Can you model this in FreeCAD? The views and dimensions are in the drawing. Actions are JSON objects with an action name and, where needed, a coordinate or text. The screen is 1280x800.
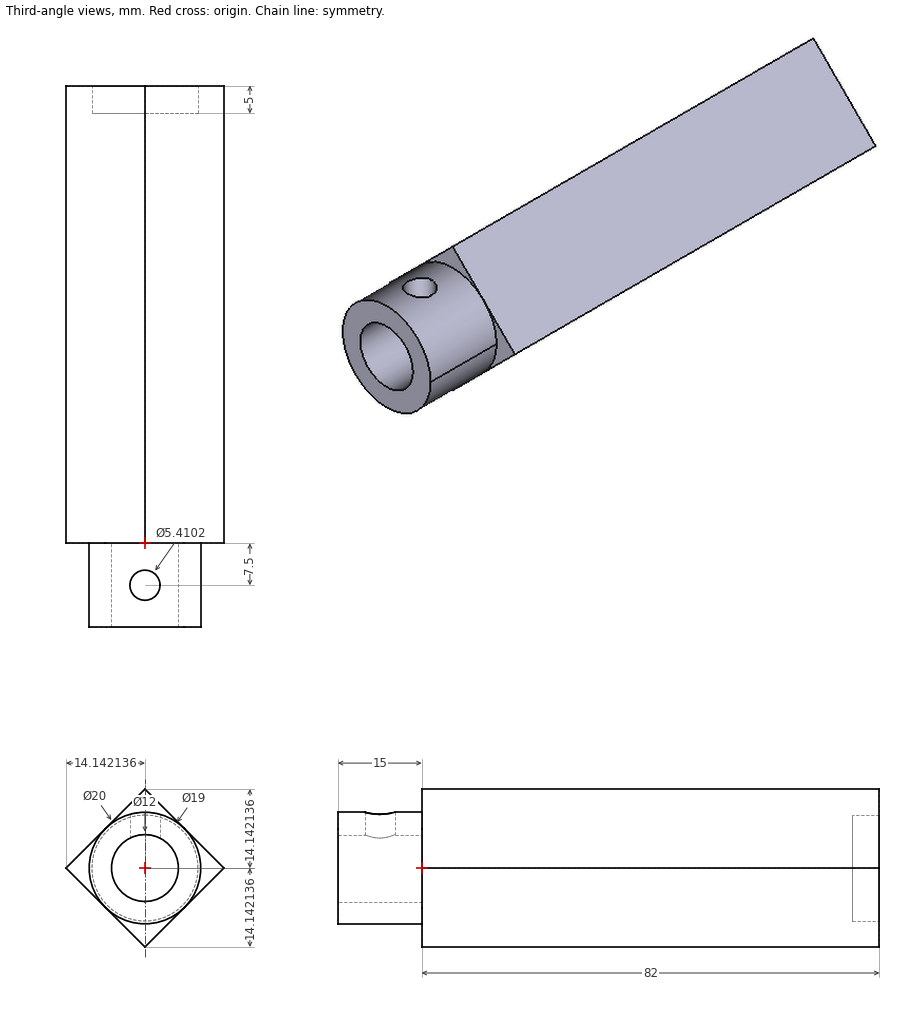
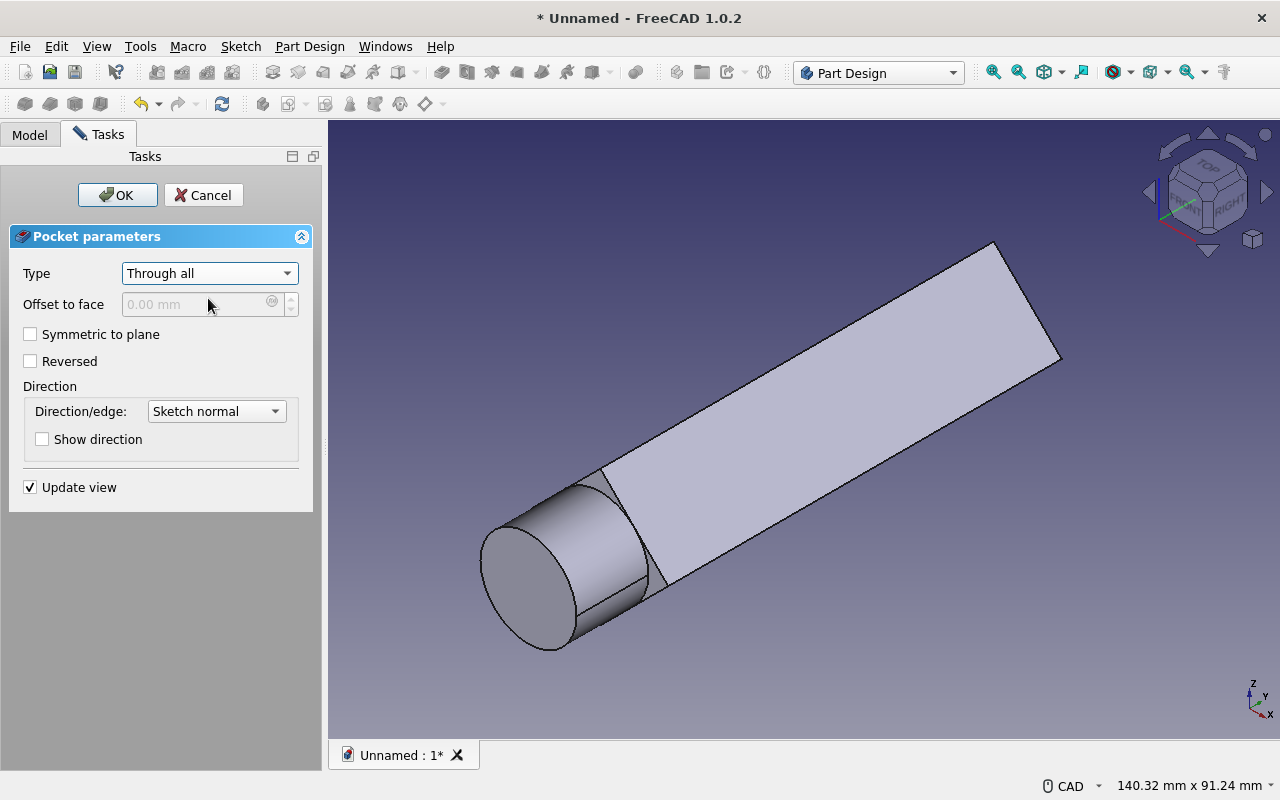
{"action": "left_click", "coordinate": [31, 361]}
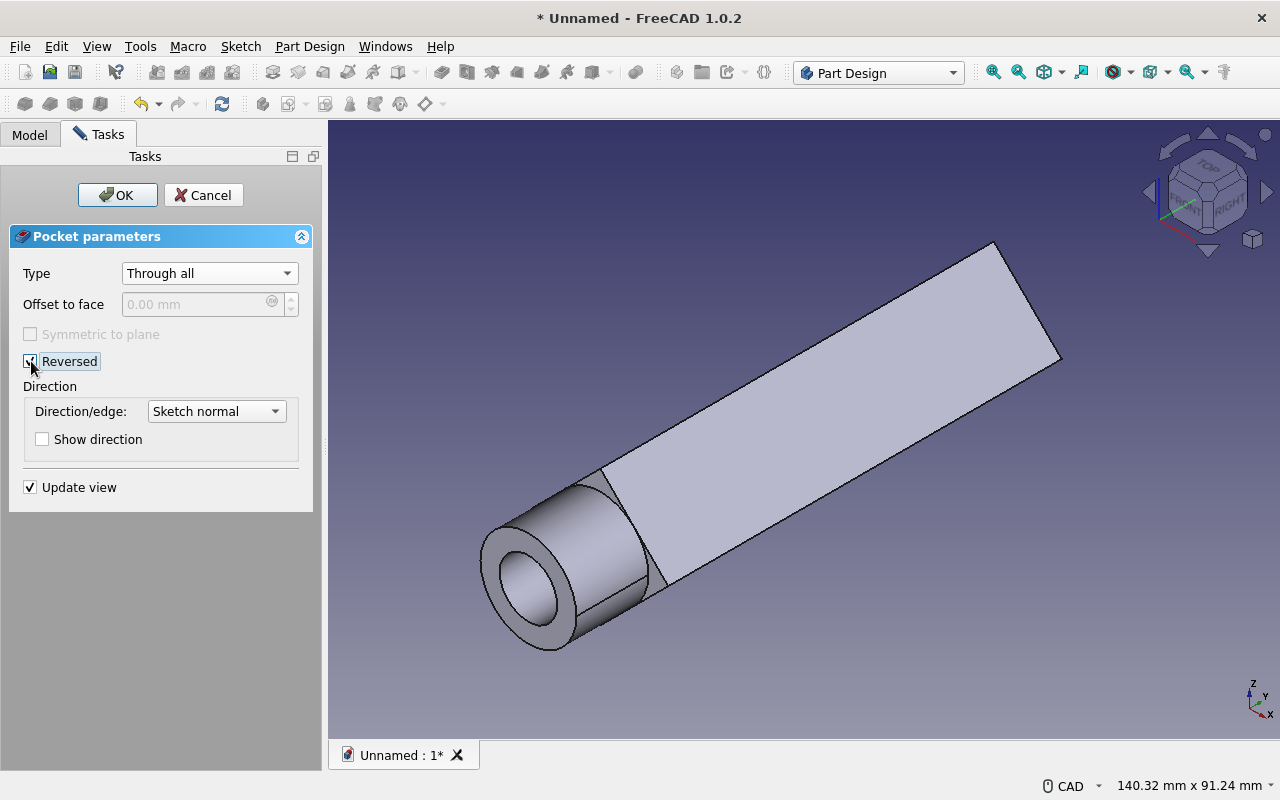
{"action": "left_click", "coordinate": [118, 195]}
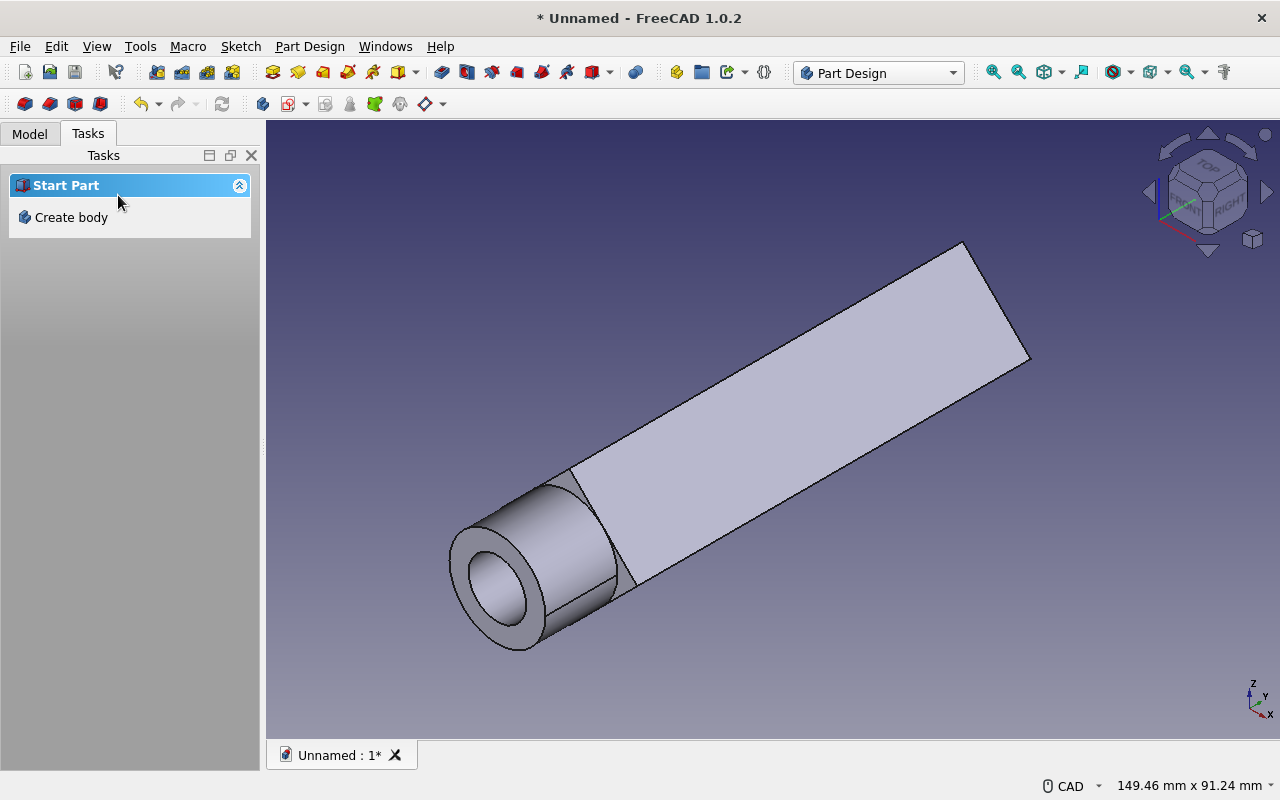
{"action": "left_click", "coordinate": [30, 134]}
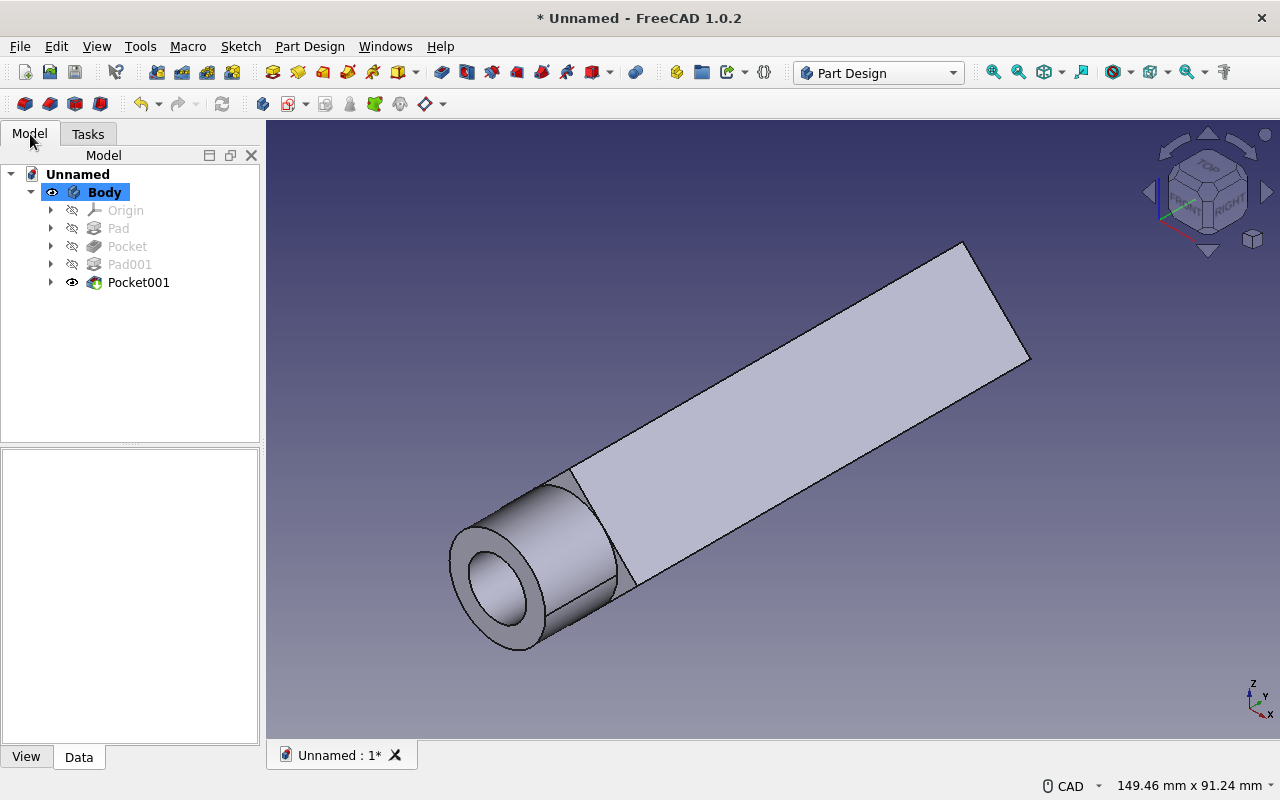
{"action": "left_click", "coordinate": [51, 210]}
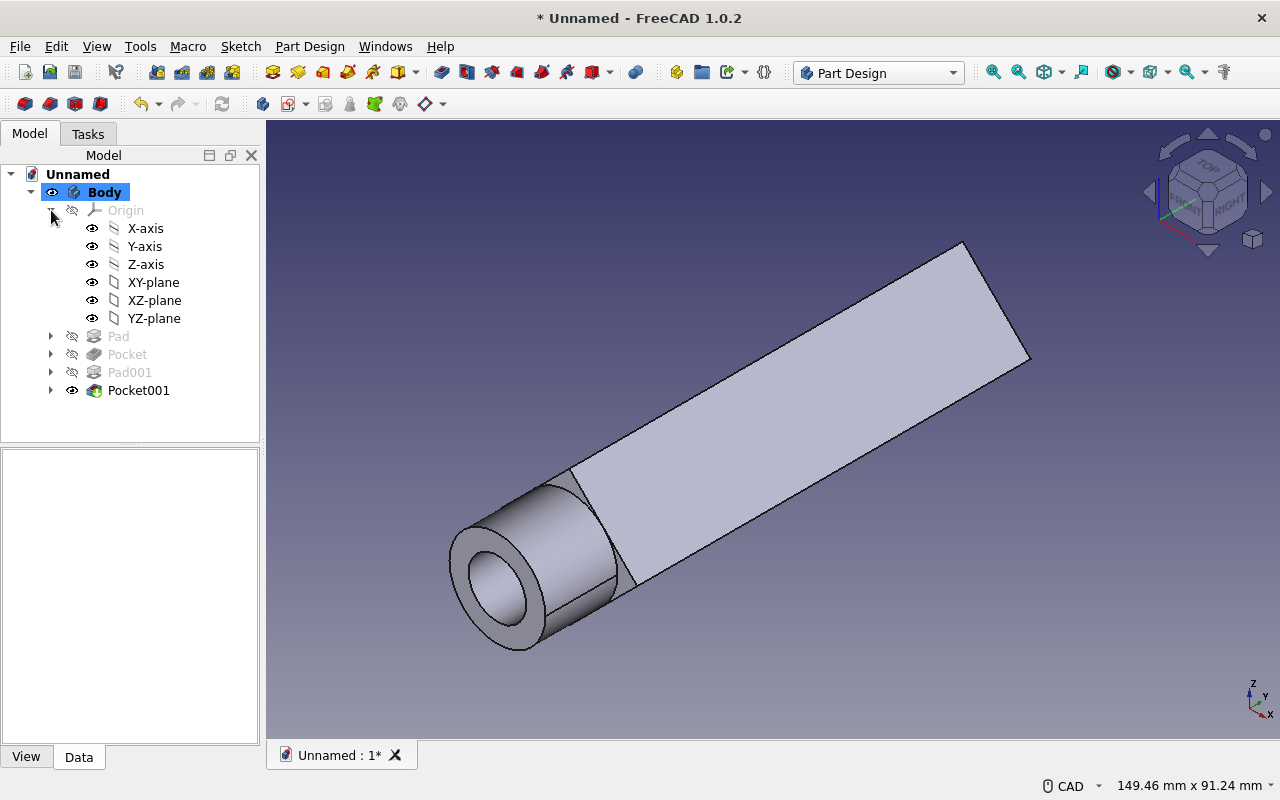
{"action": "left_click", "coordinate": [137, 282]}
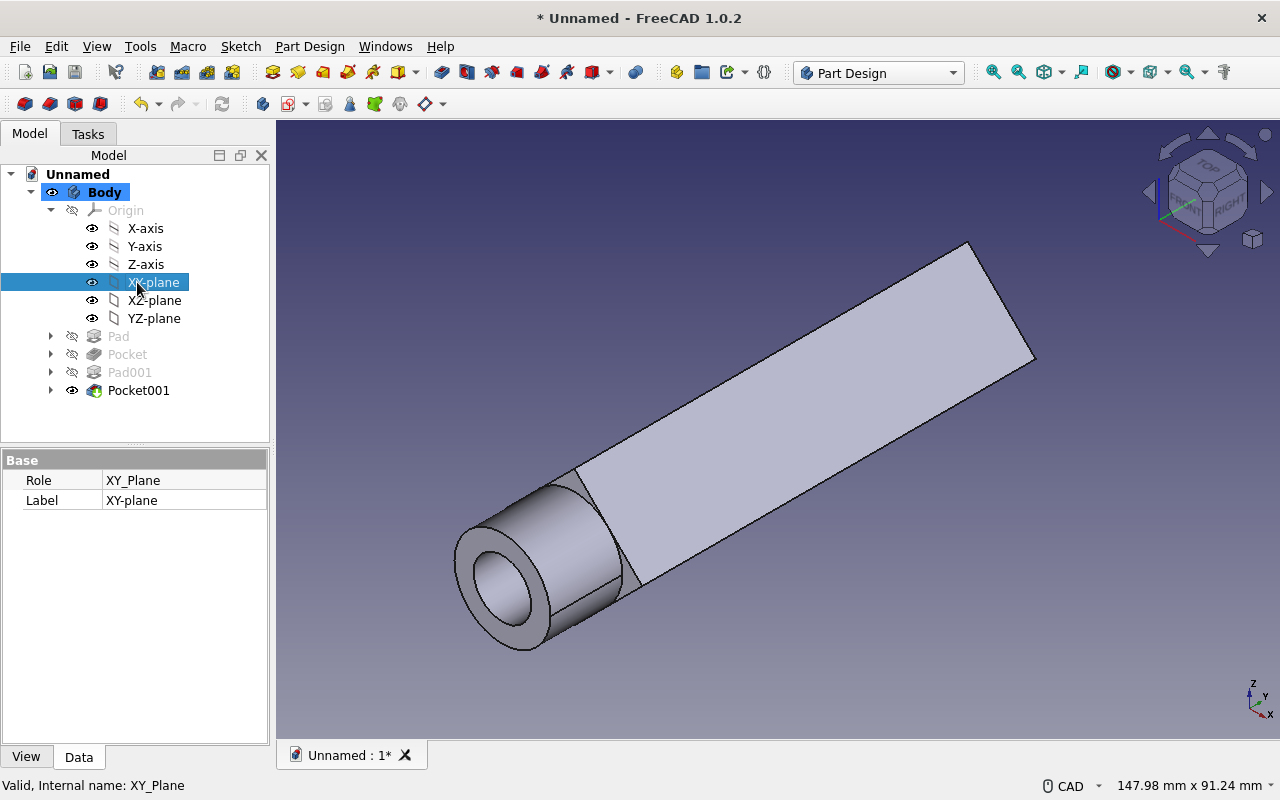
{"action": "left_click", "coordinate": [424, 104]}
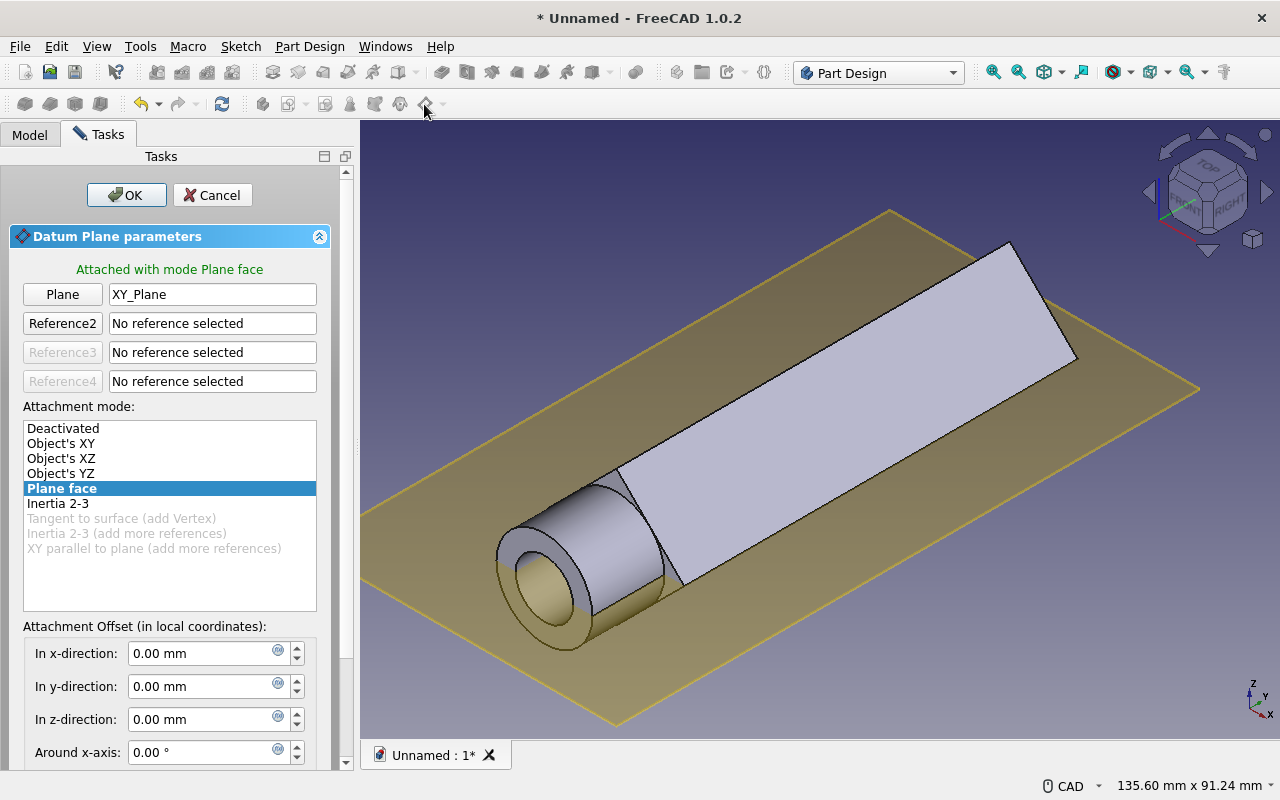
{"action": "triple_click", "coordinate": [210, 720]}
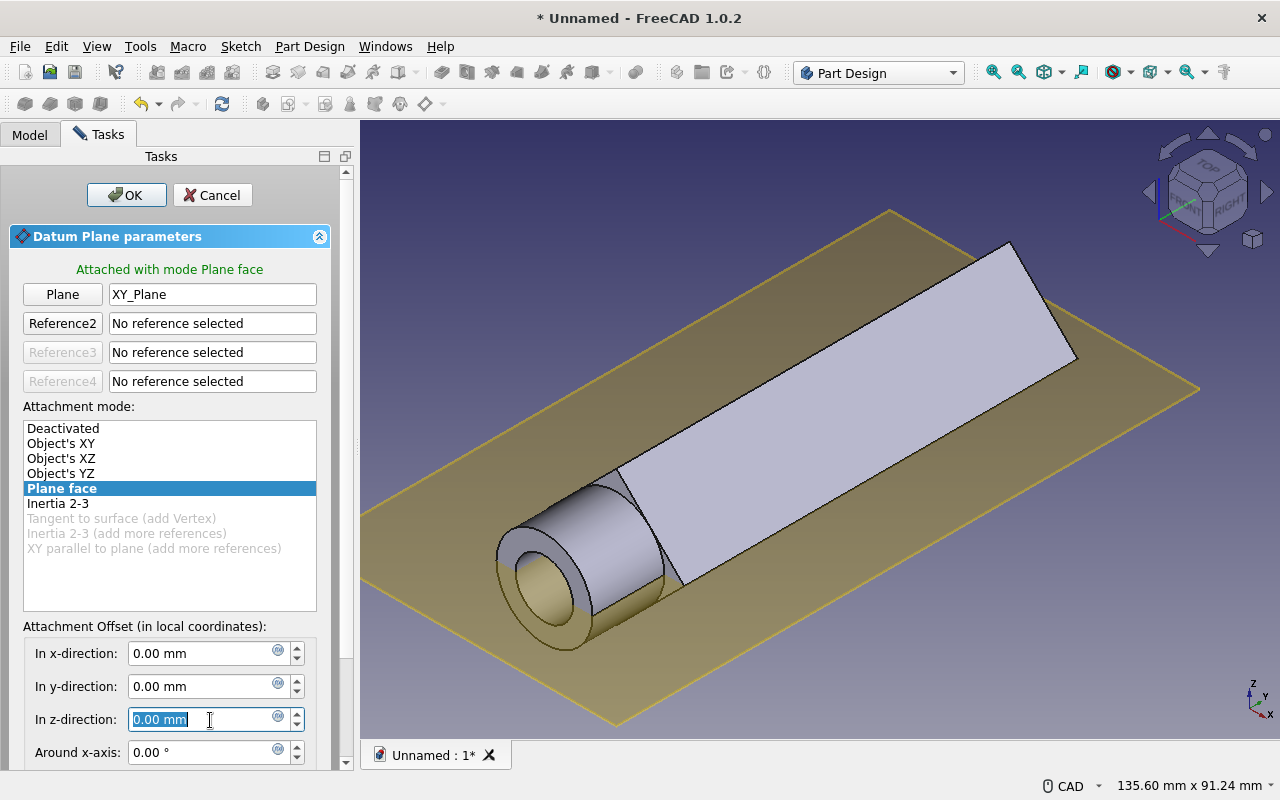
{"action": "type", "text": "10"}
{"action": "key", "text": "Tab"}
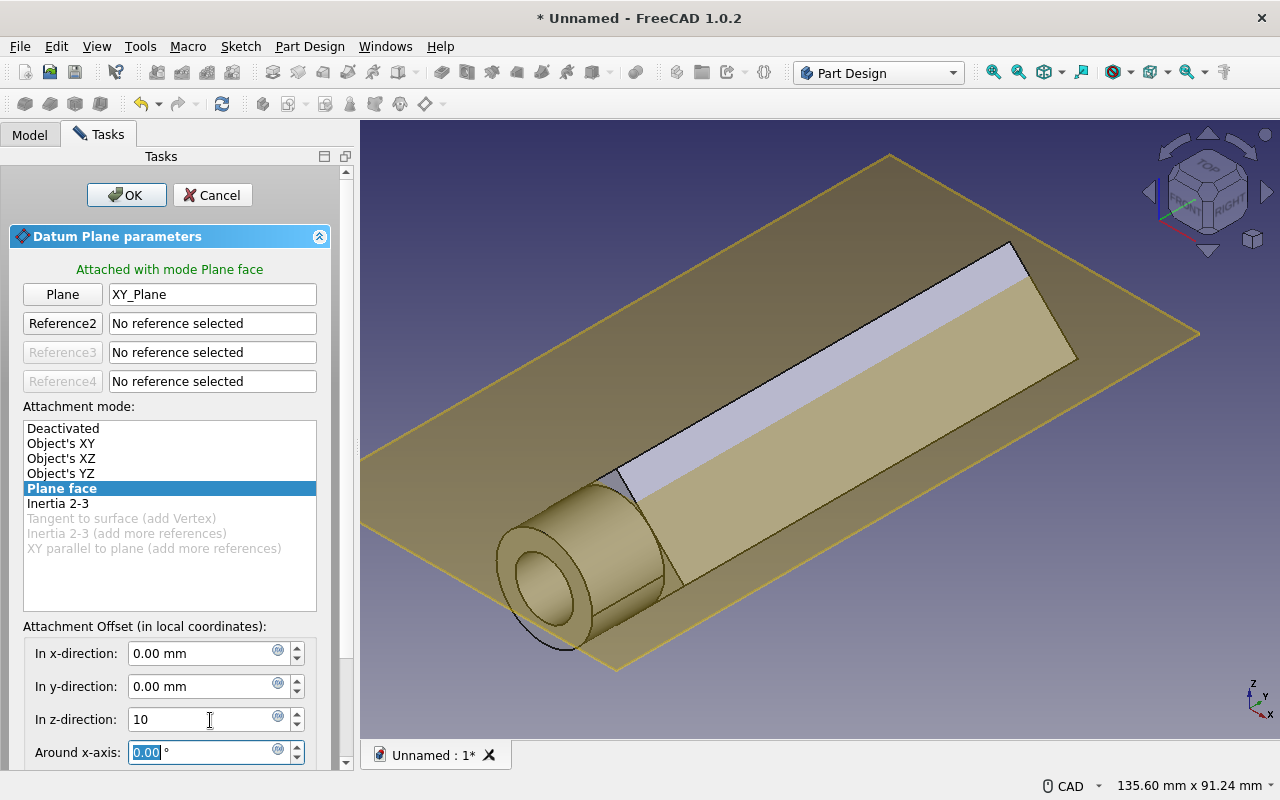
{"action": "left_click", "coordinate": [127, 195]}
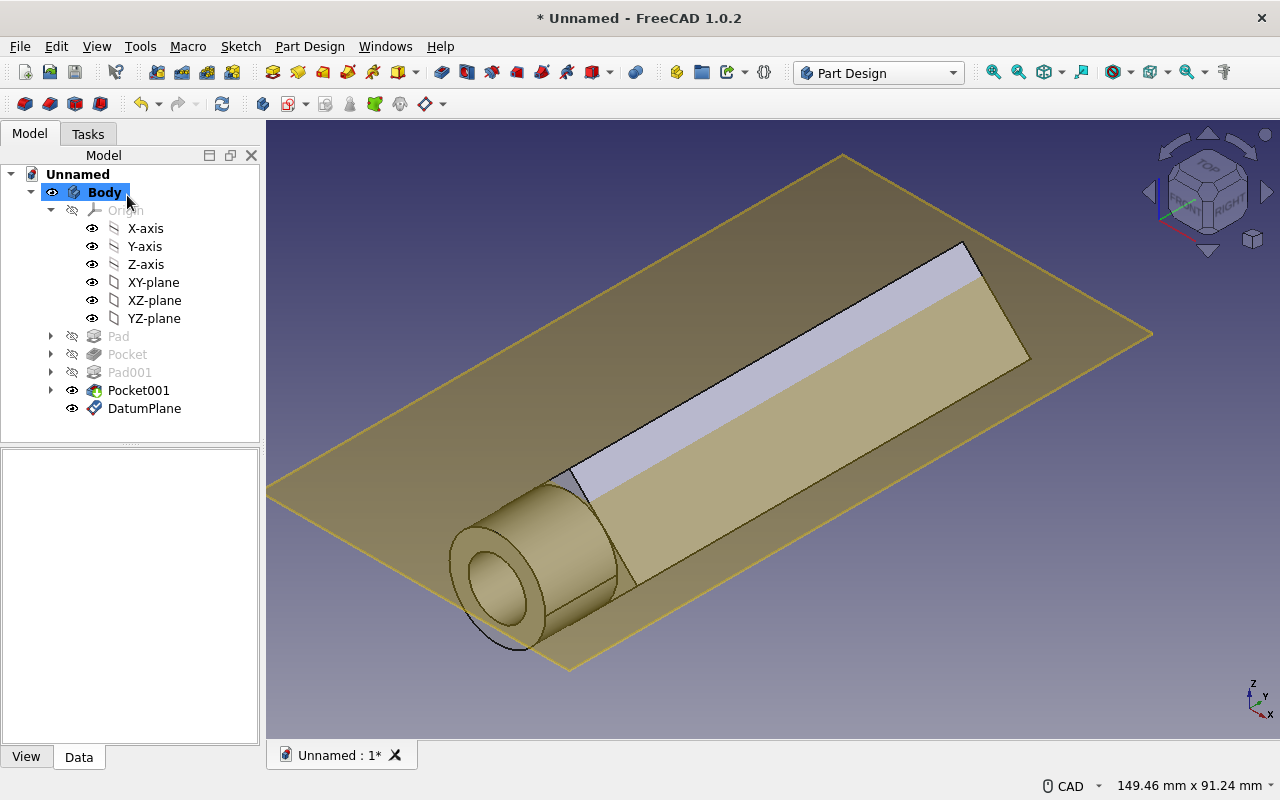
{"action": "left_click", "coordinate": [117, 408]}